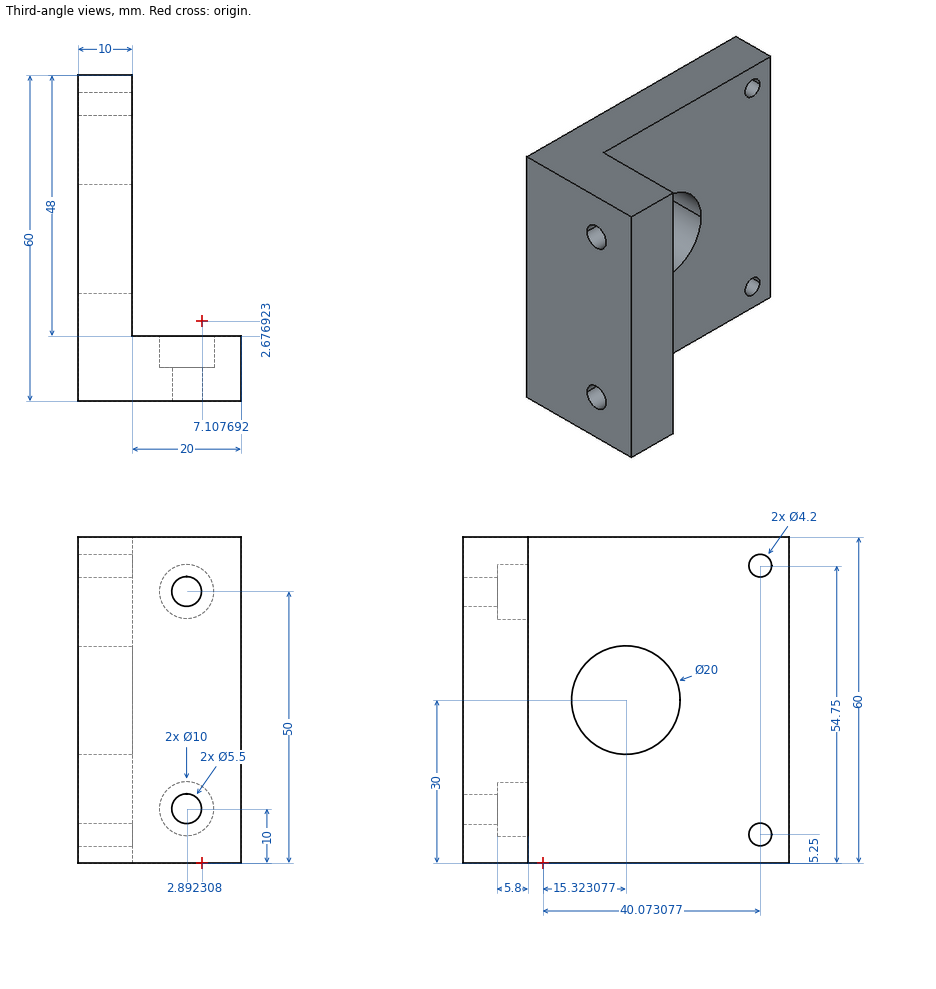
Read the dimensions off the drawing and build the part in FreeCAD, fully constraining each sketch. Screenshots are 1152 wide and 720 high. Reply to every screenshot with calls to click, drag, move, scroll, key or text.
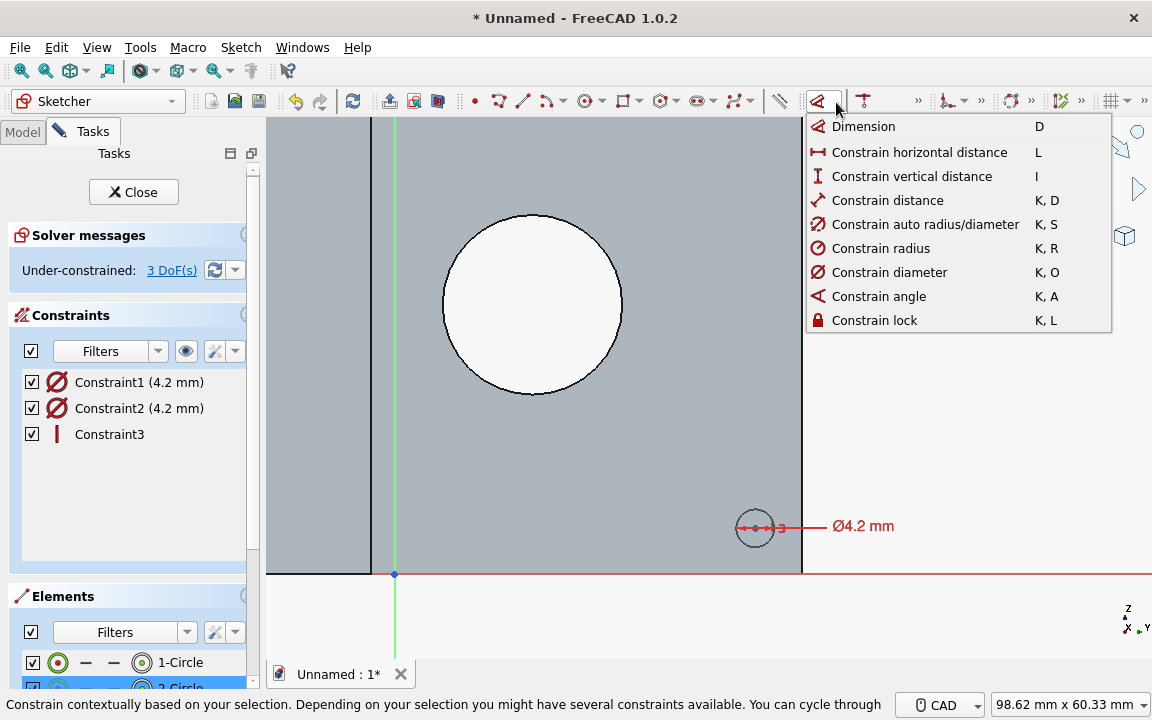
click(959, 176)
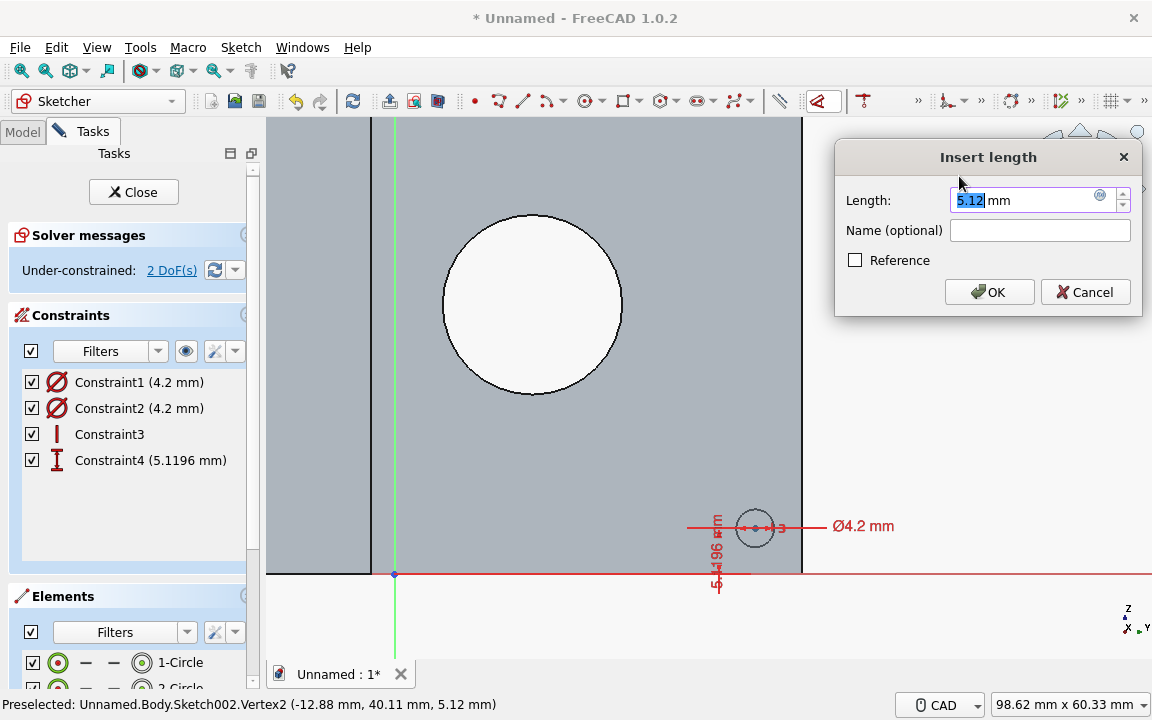
text(5.25)
key(Return)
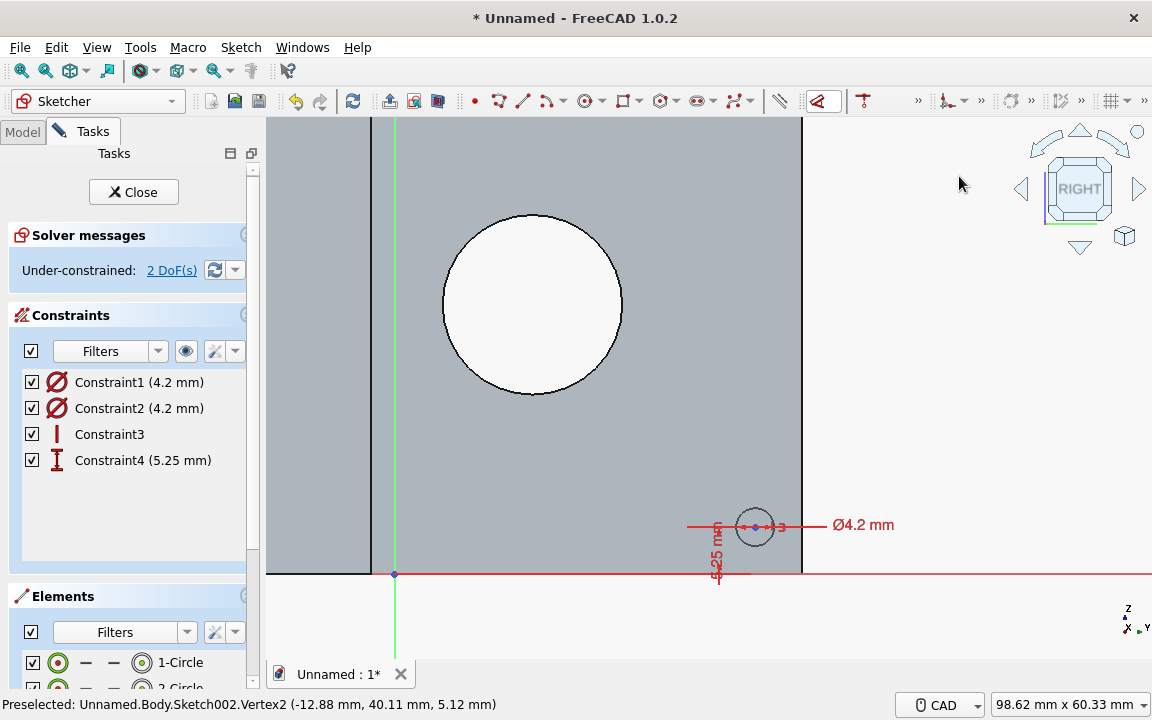
scroll(755, 528, down, 2)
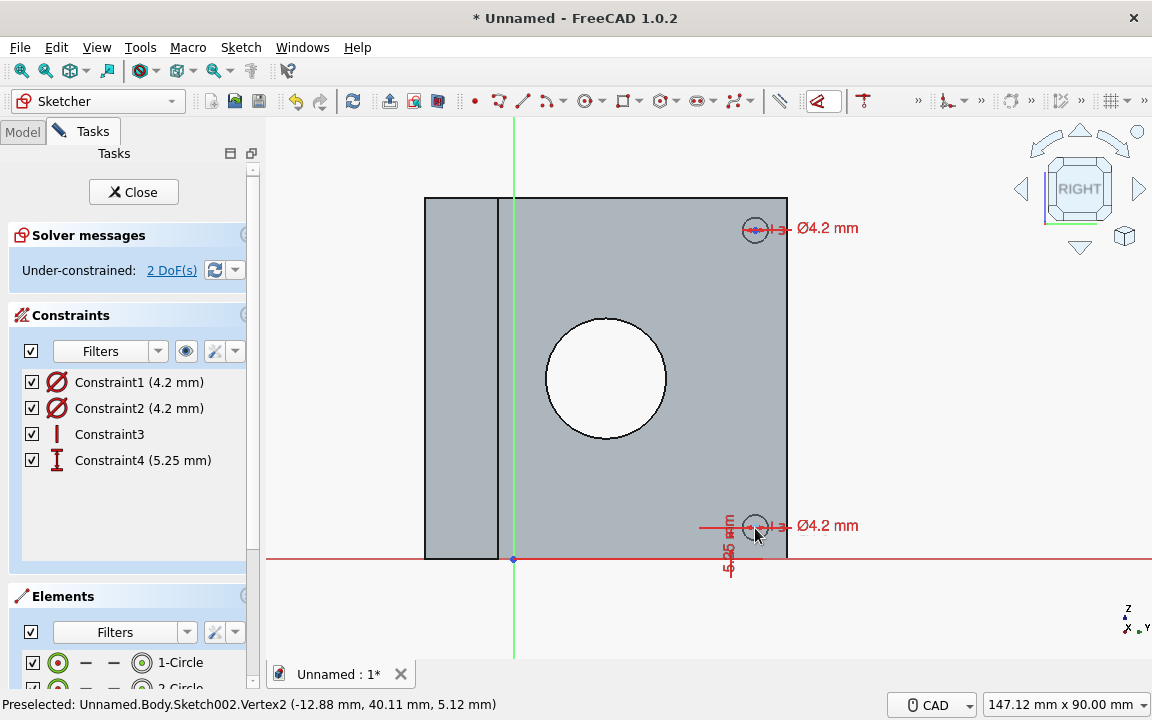
click(755, 230)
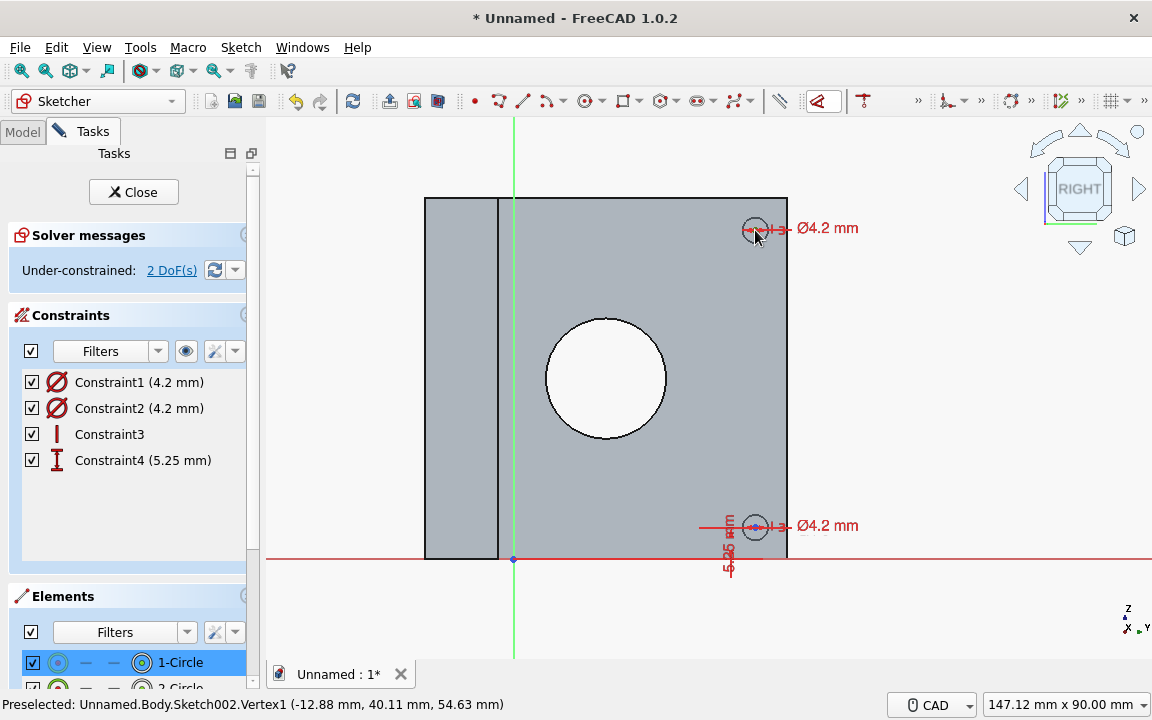
click(836, 102)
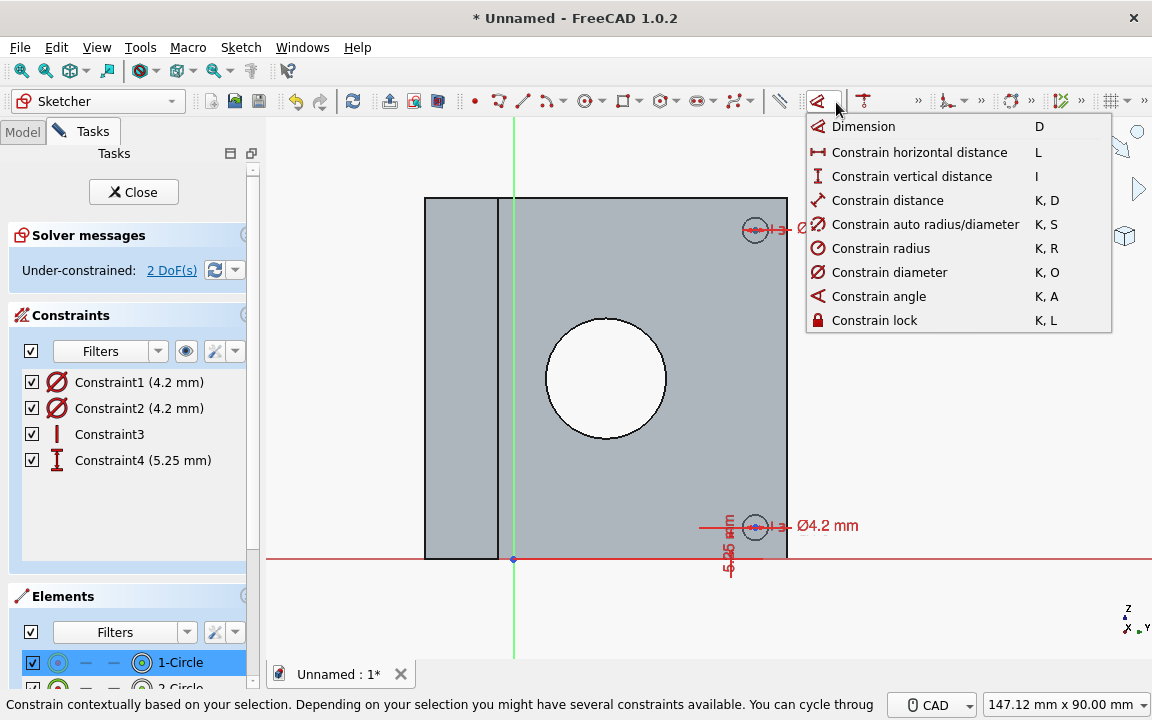
click(959, 176)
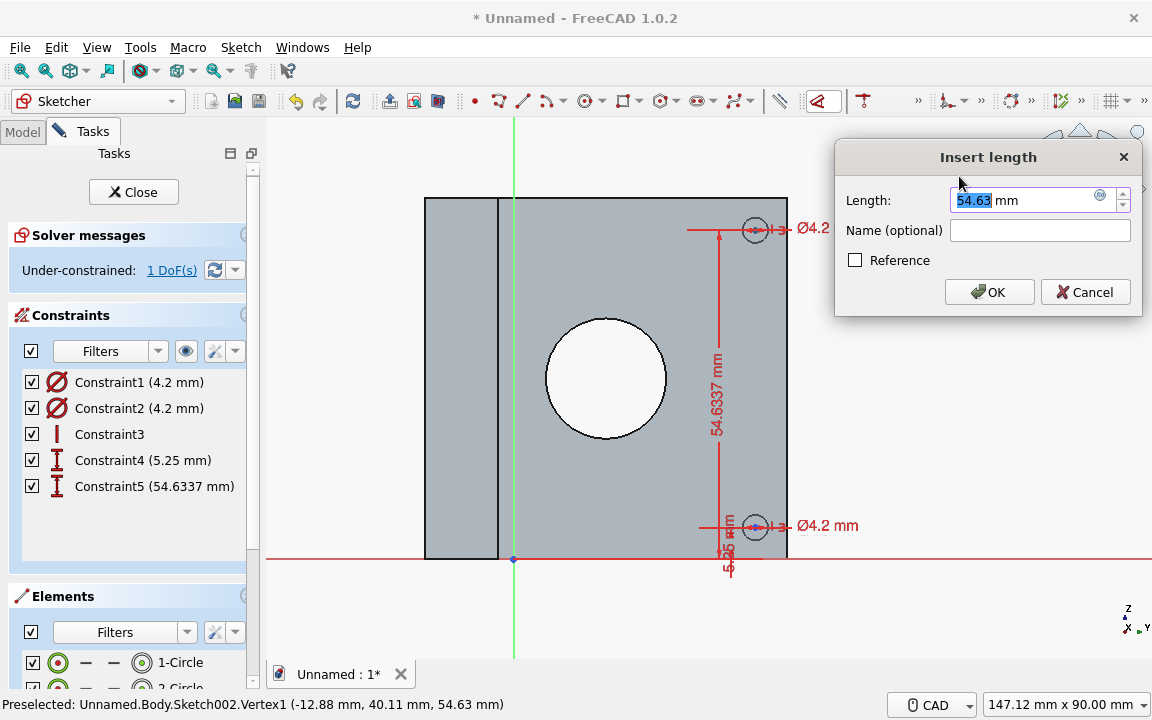
text(54.75)
key(Return)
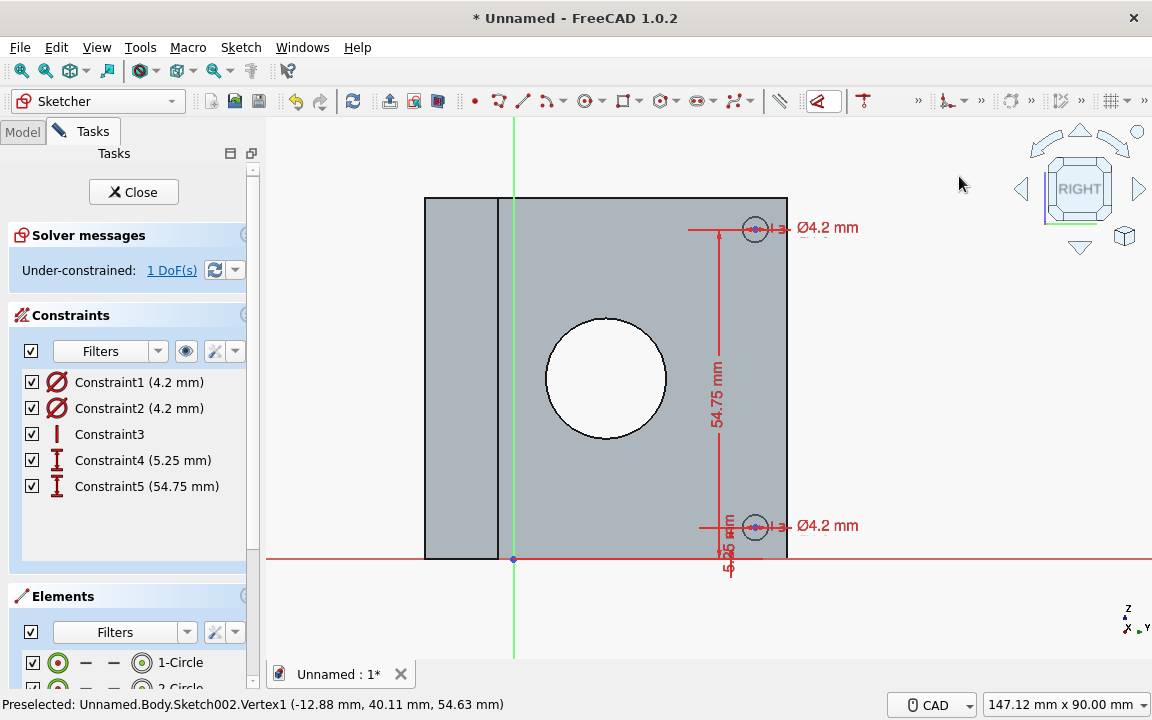
click(755, 230)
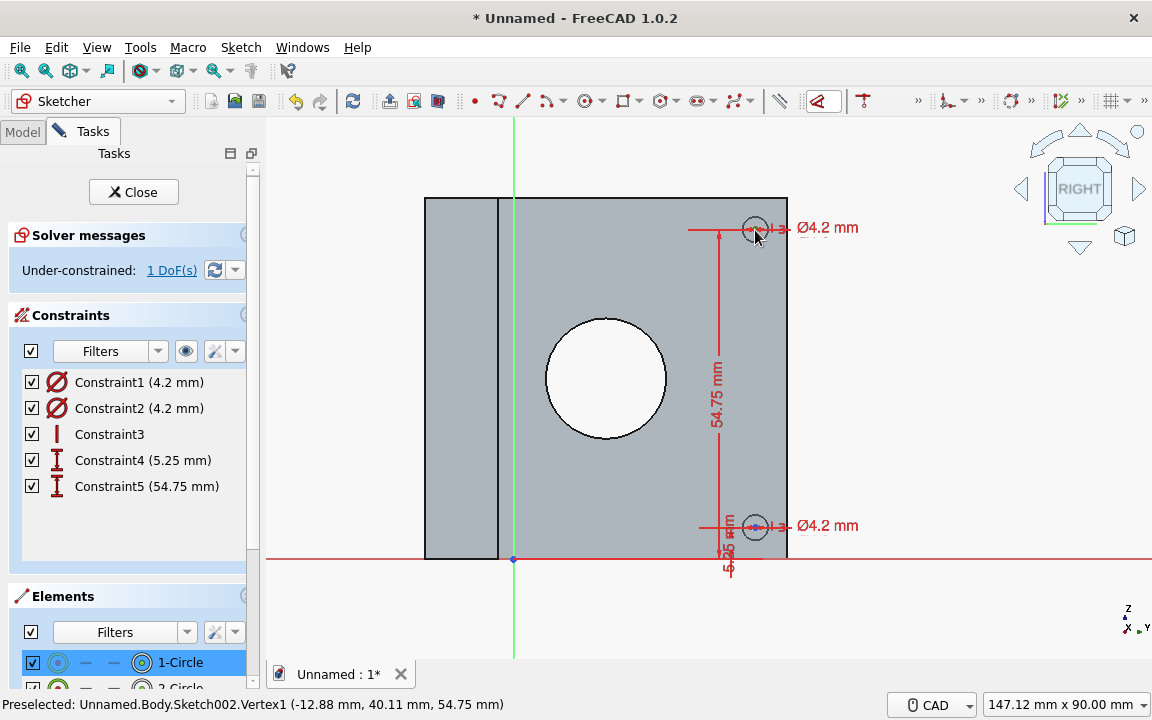
key(l)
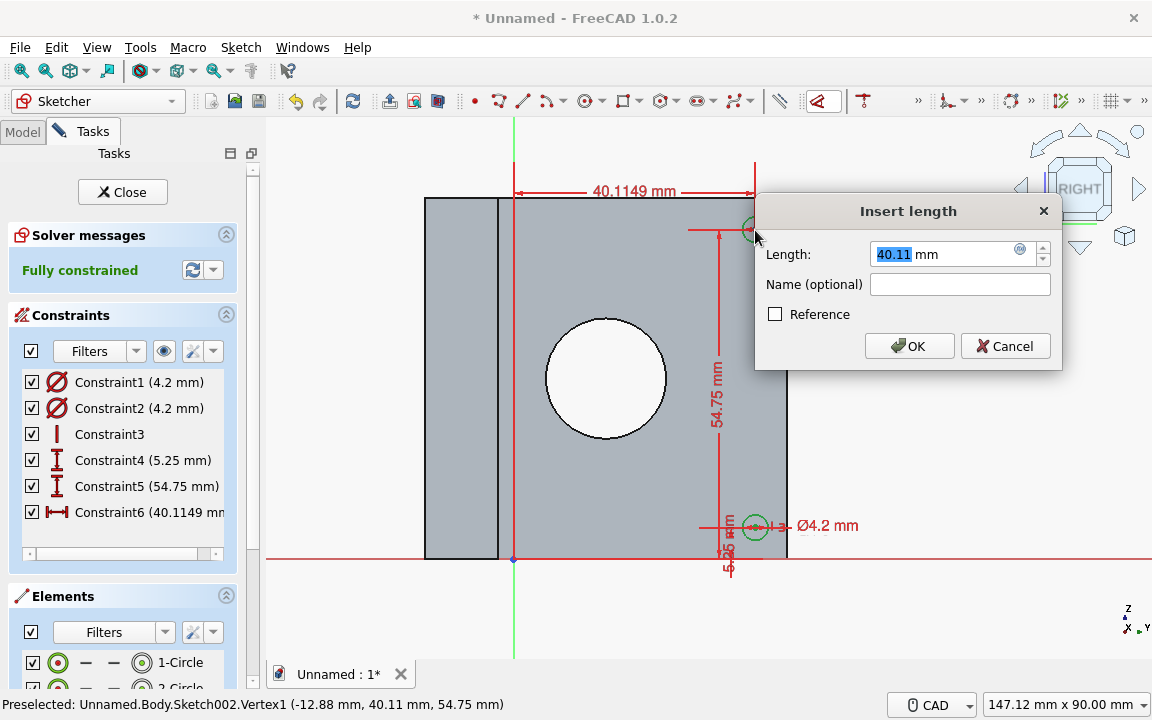
text(40.073077)
key(Return)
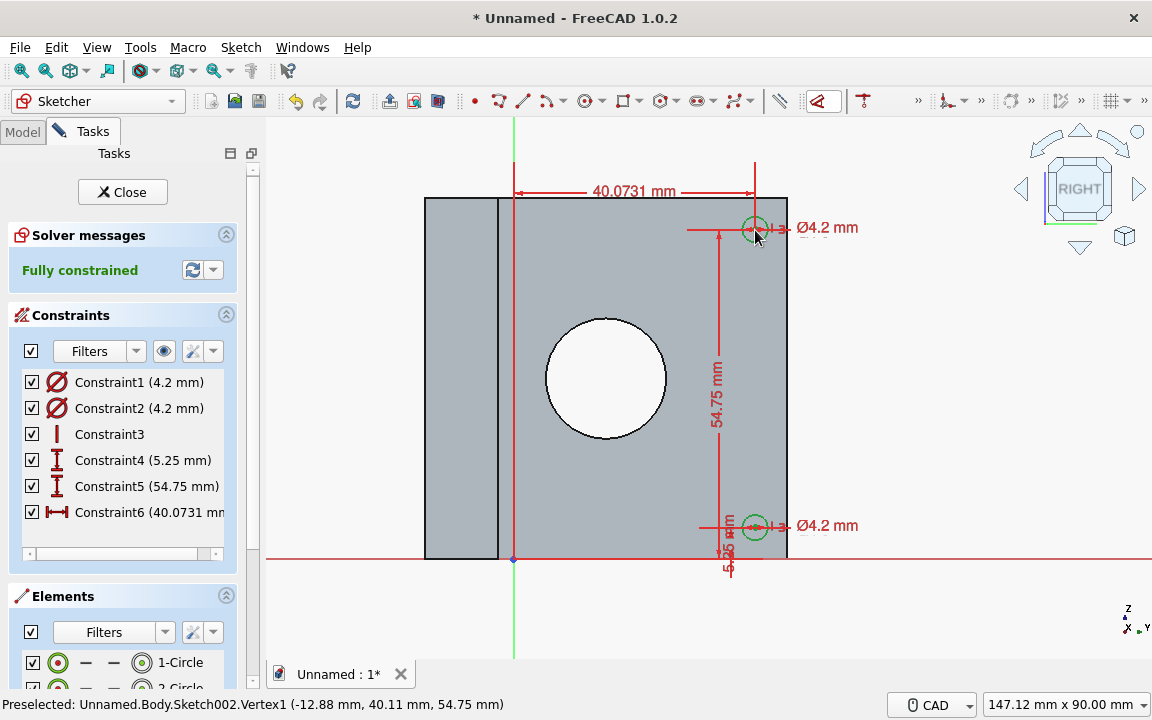
click(123, 192)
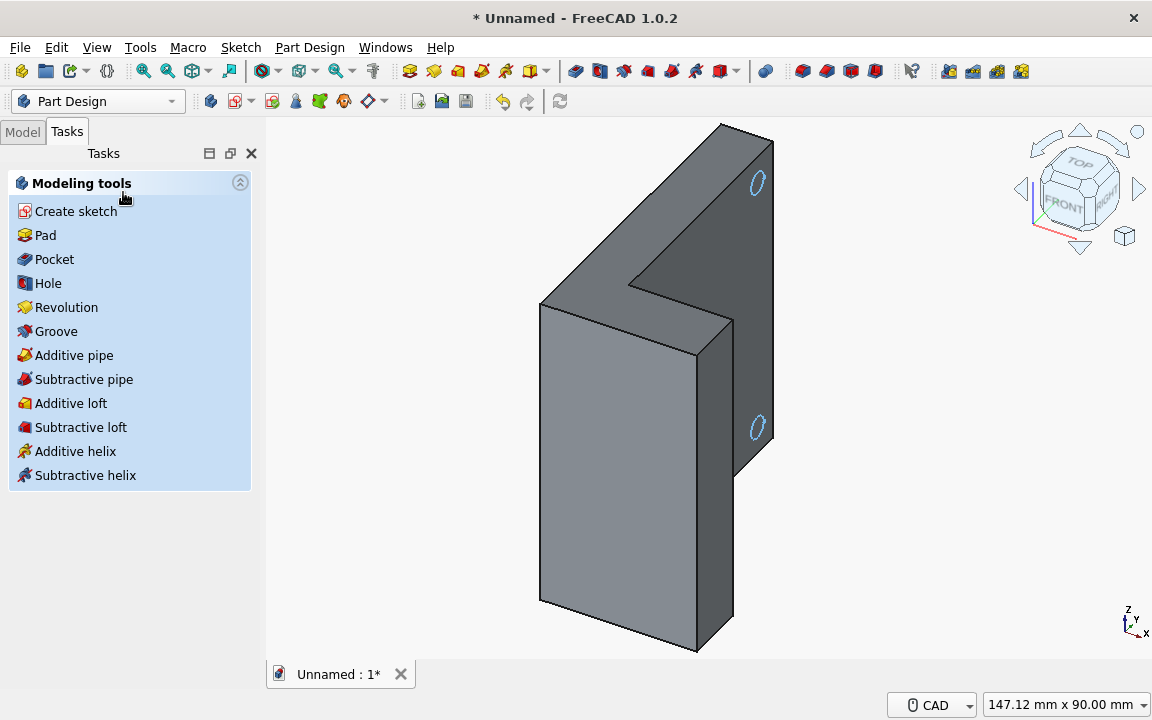
click(576, 72)